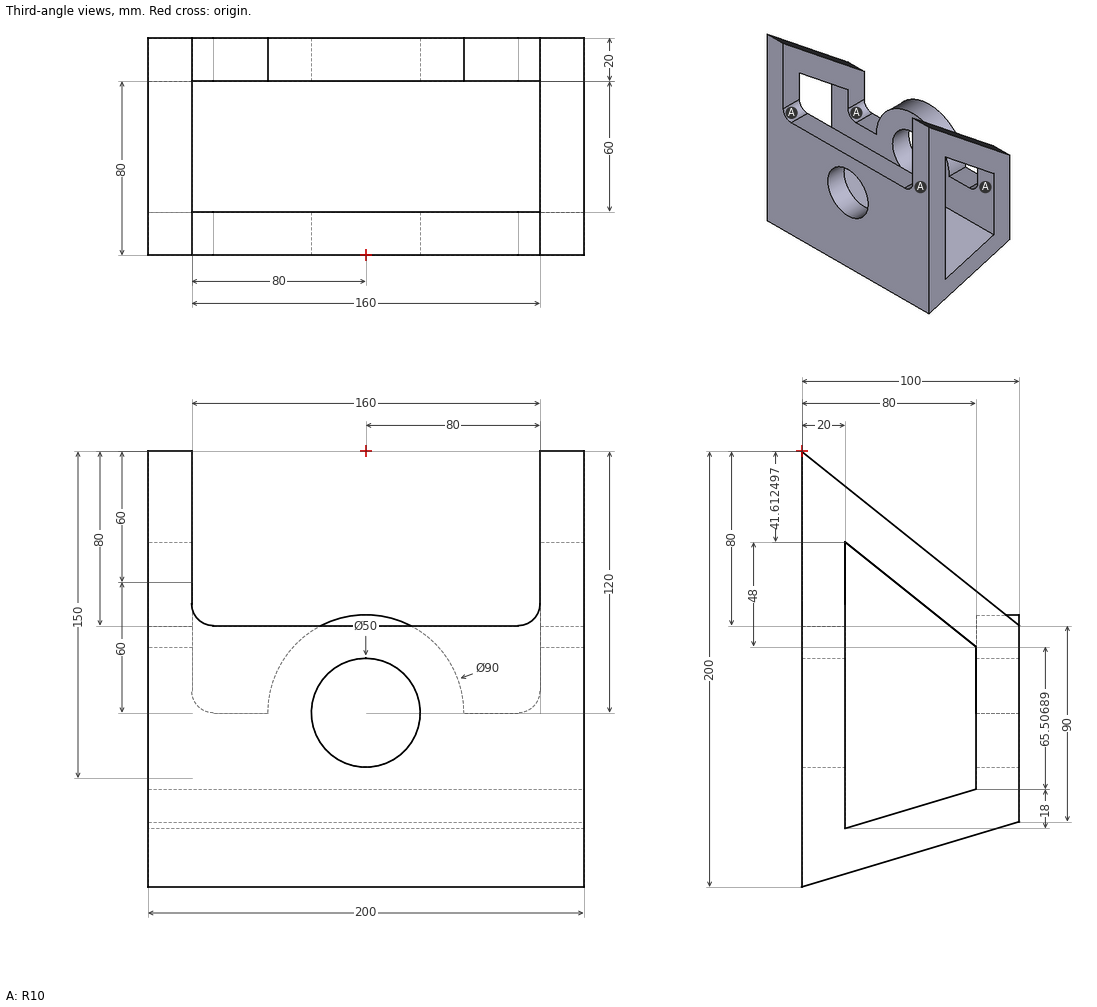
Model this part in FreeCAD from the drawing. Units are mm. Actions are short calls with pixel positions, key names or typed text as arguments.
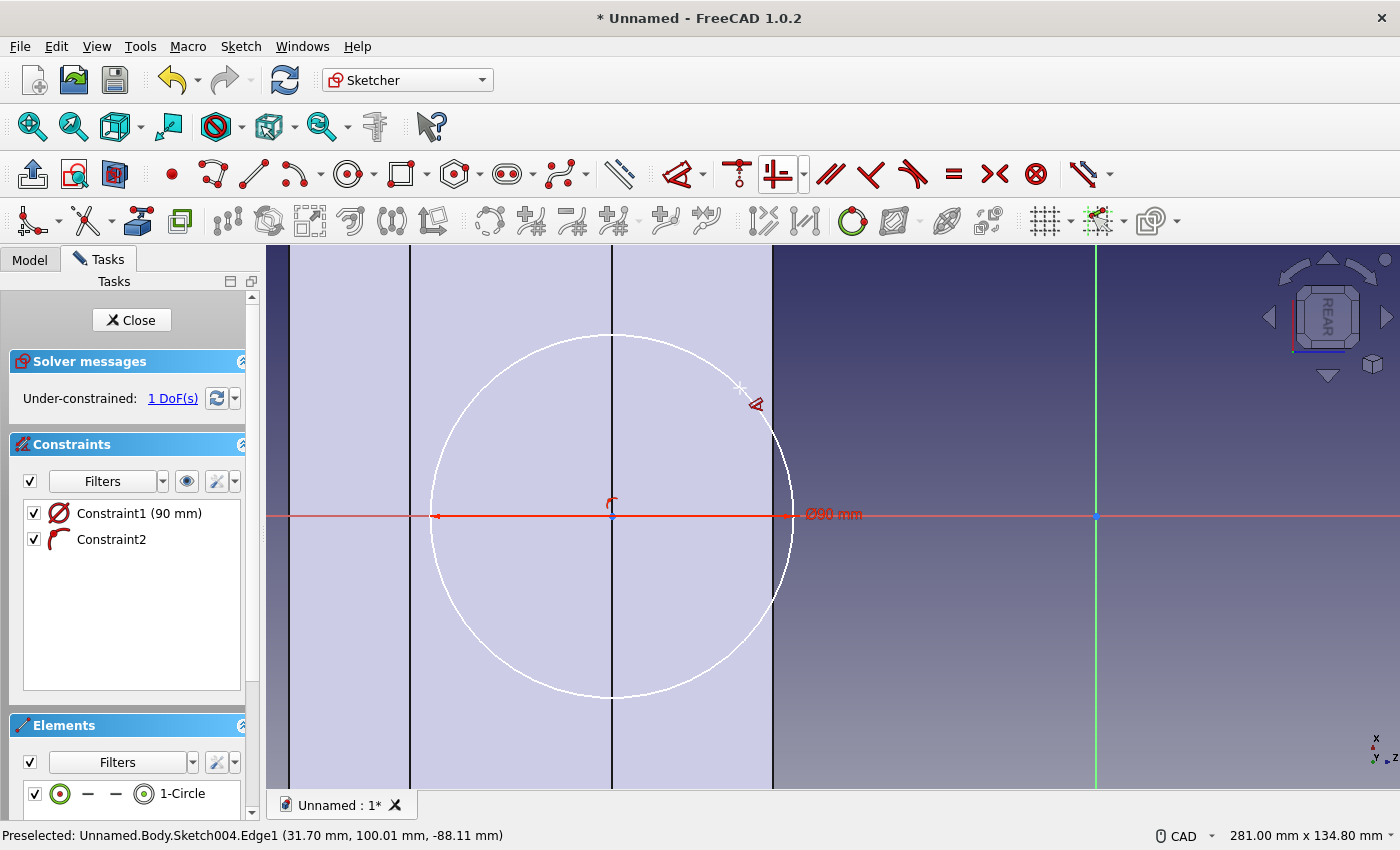
click(612, 516)
click(854, 550)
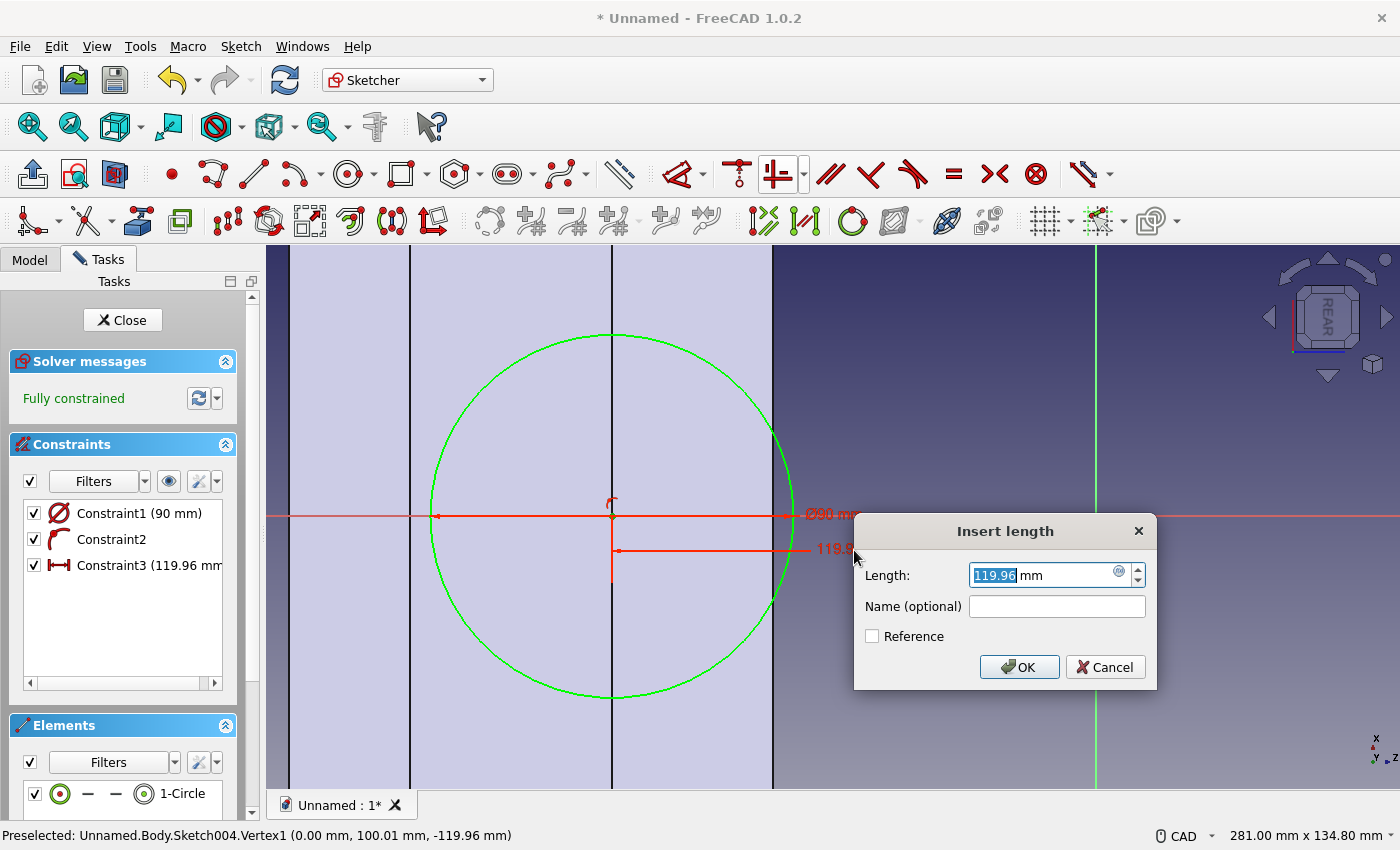
text(120)
key(Return)
key(Escape)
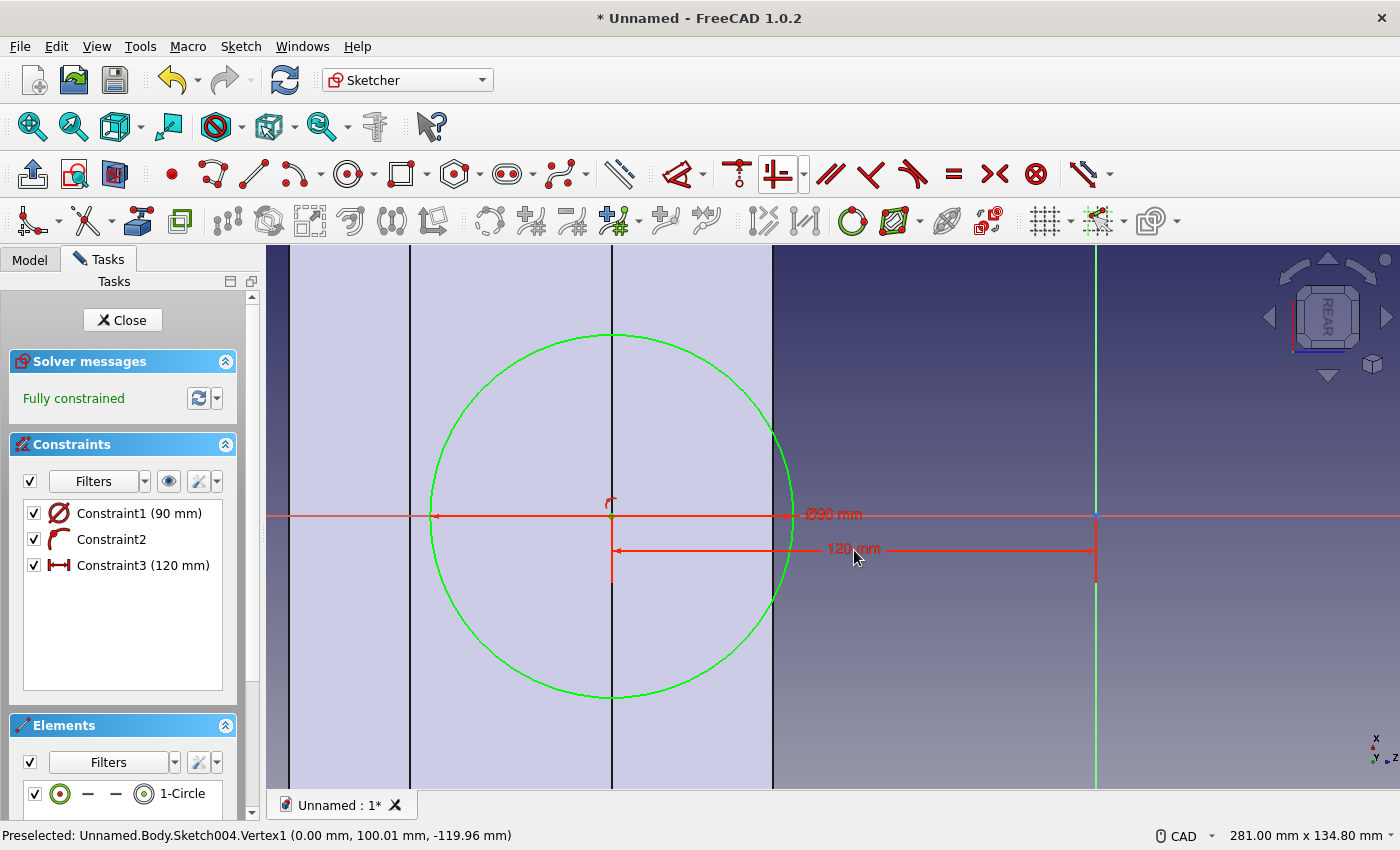
click(123, 320)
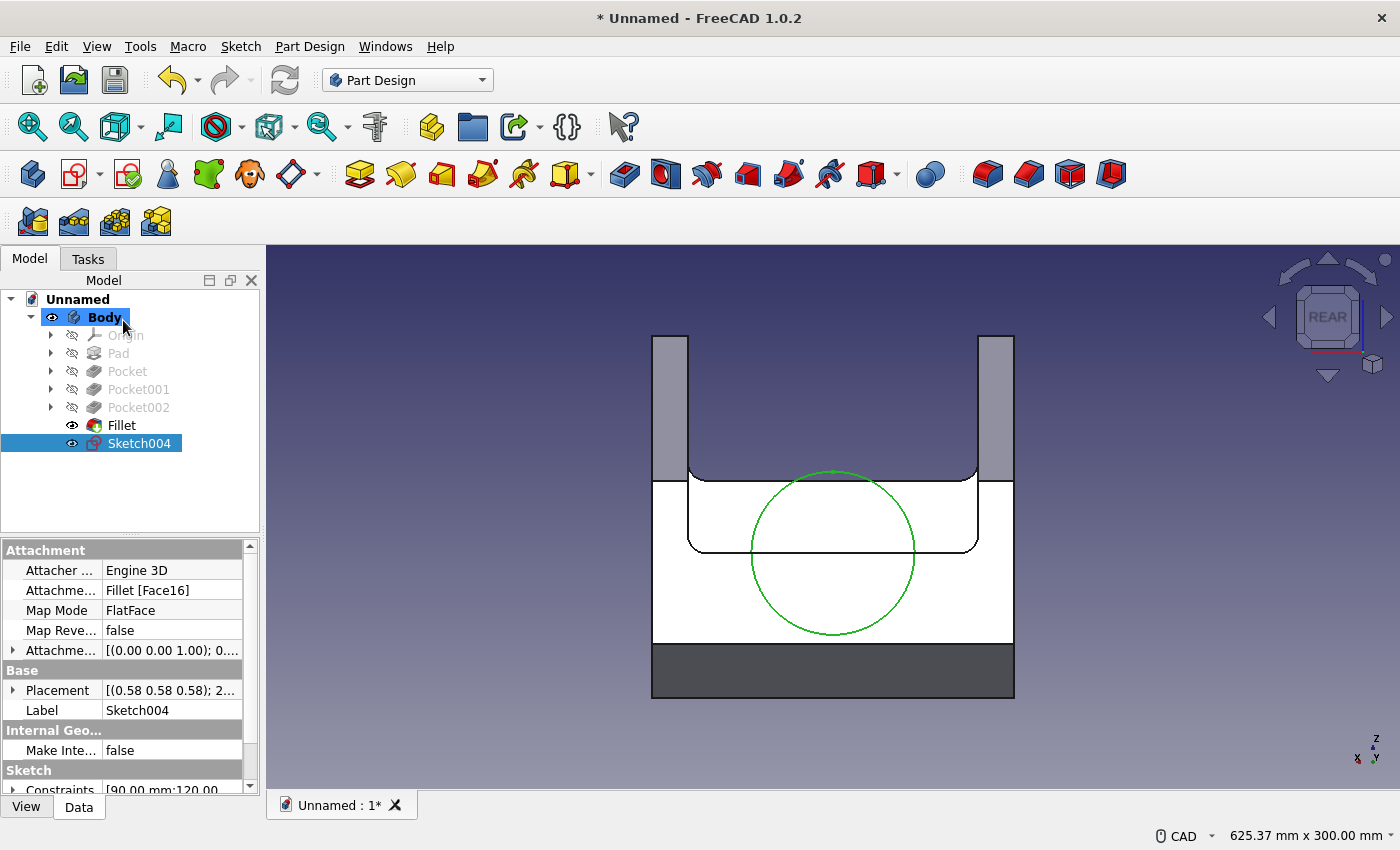
click(360, 174)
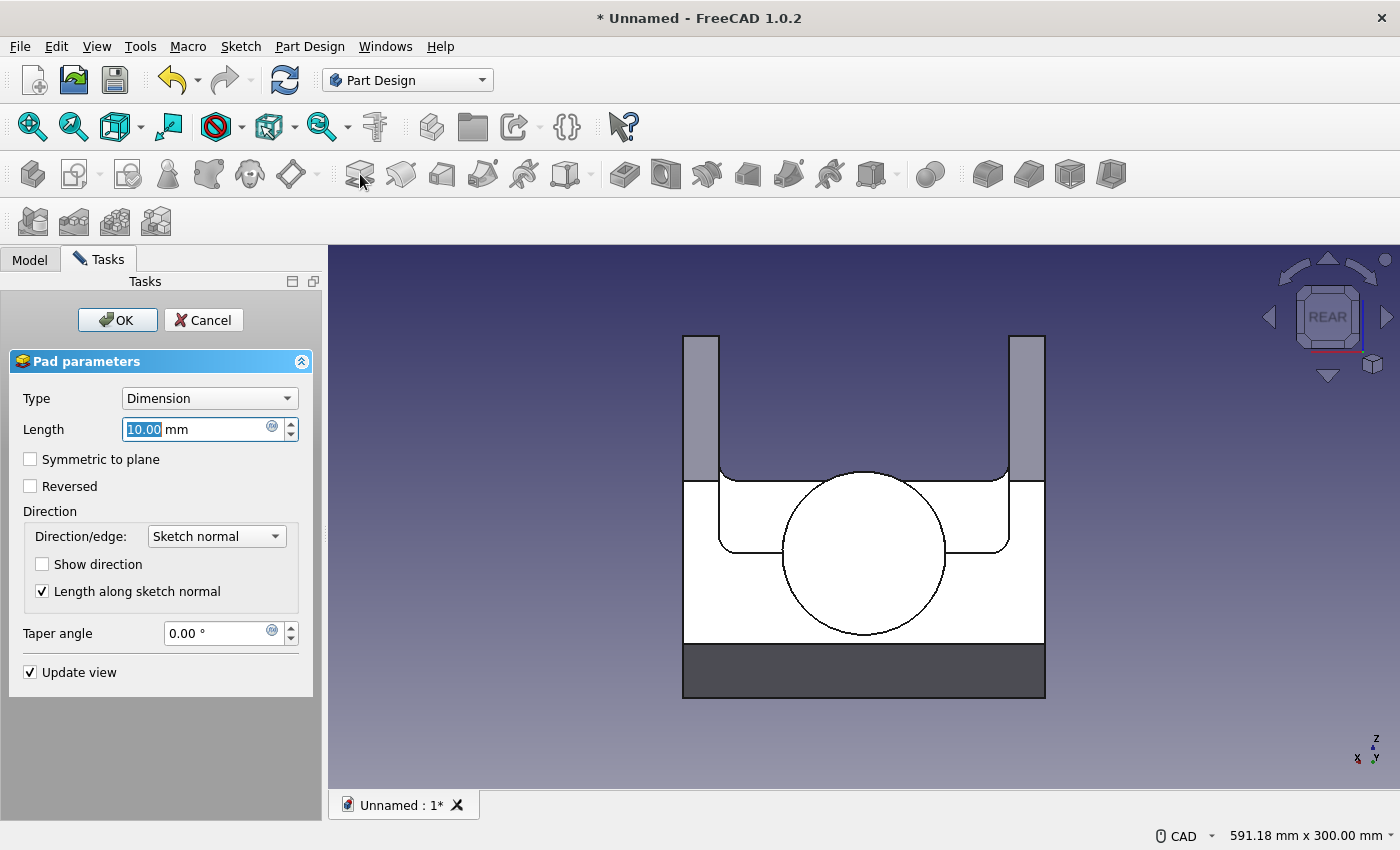
text(20)
key(Tab)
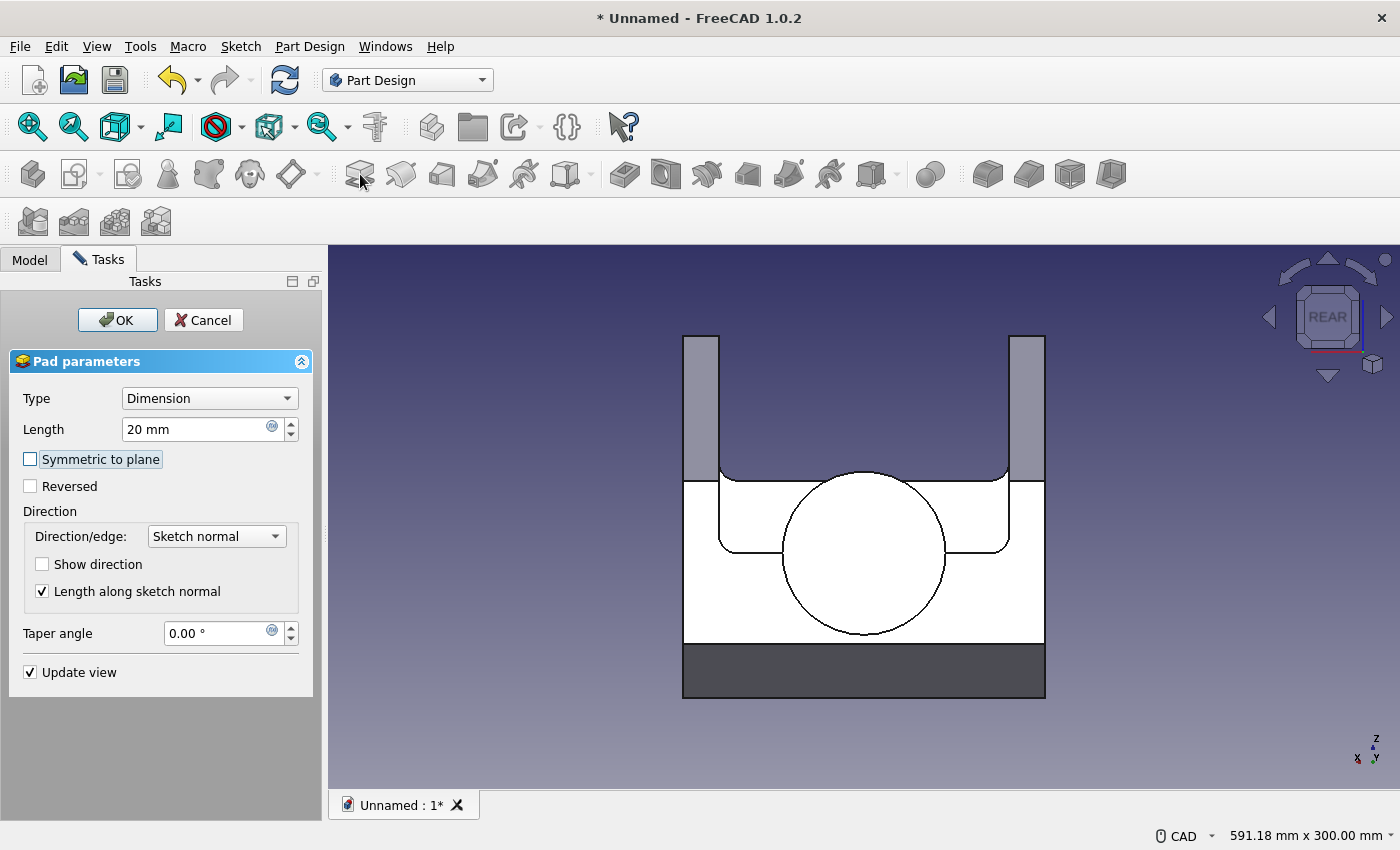
click(31, 486)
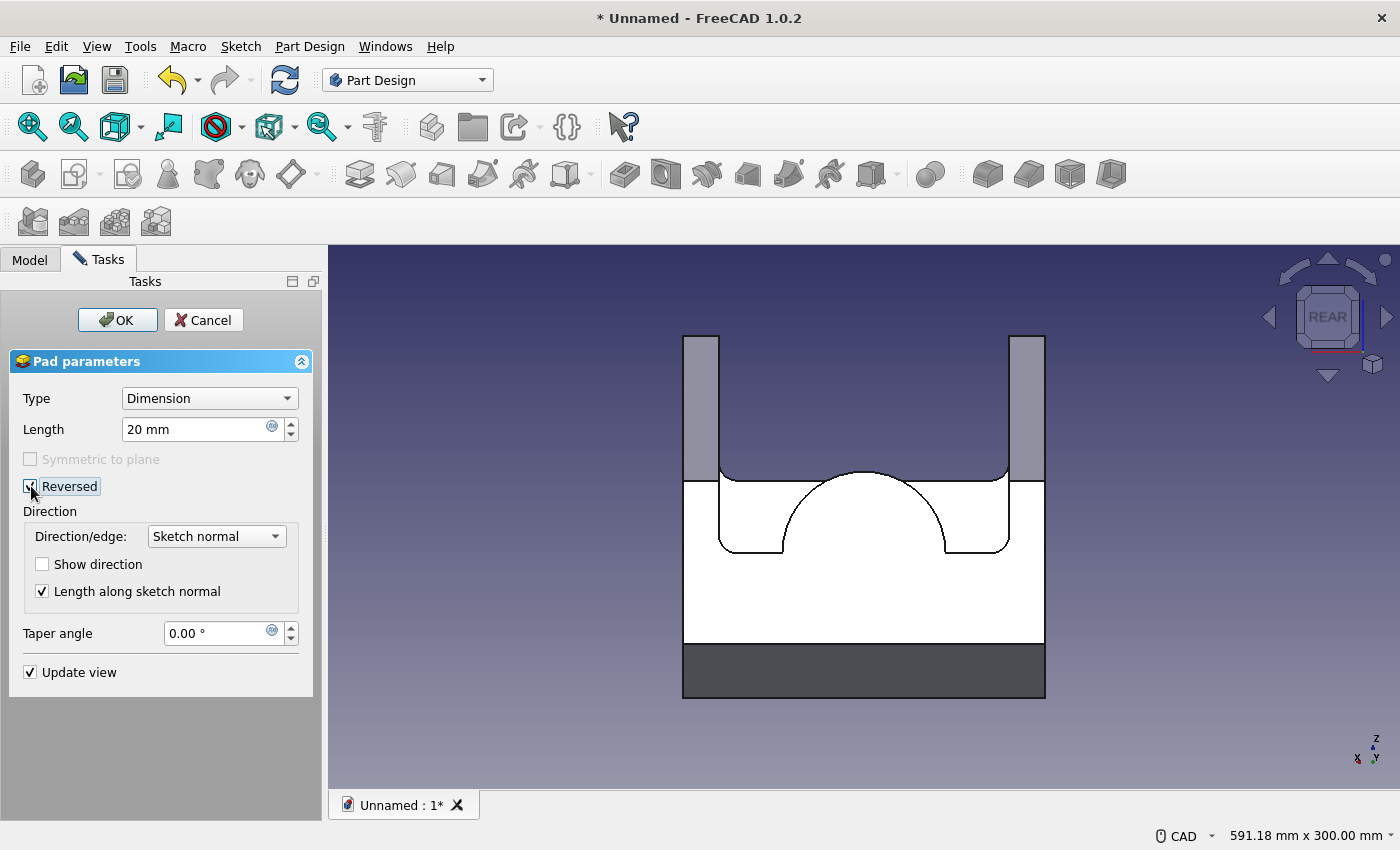
click(118, 320)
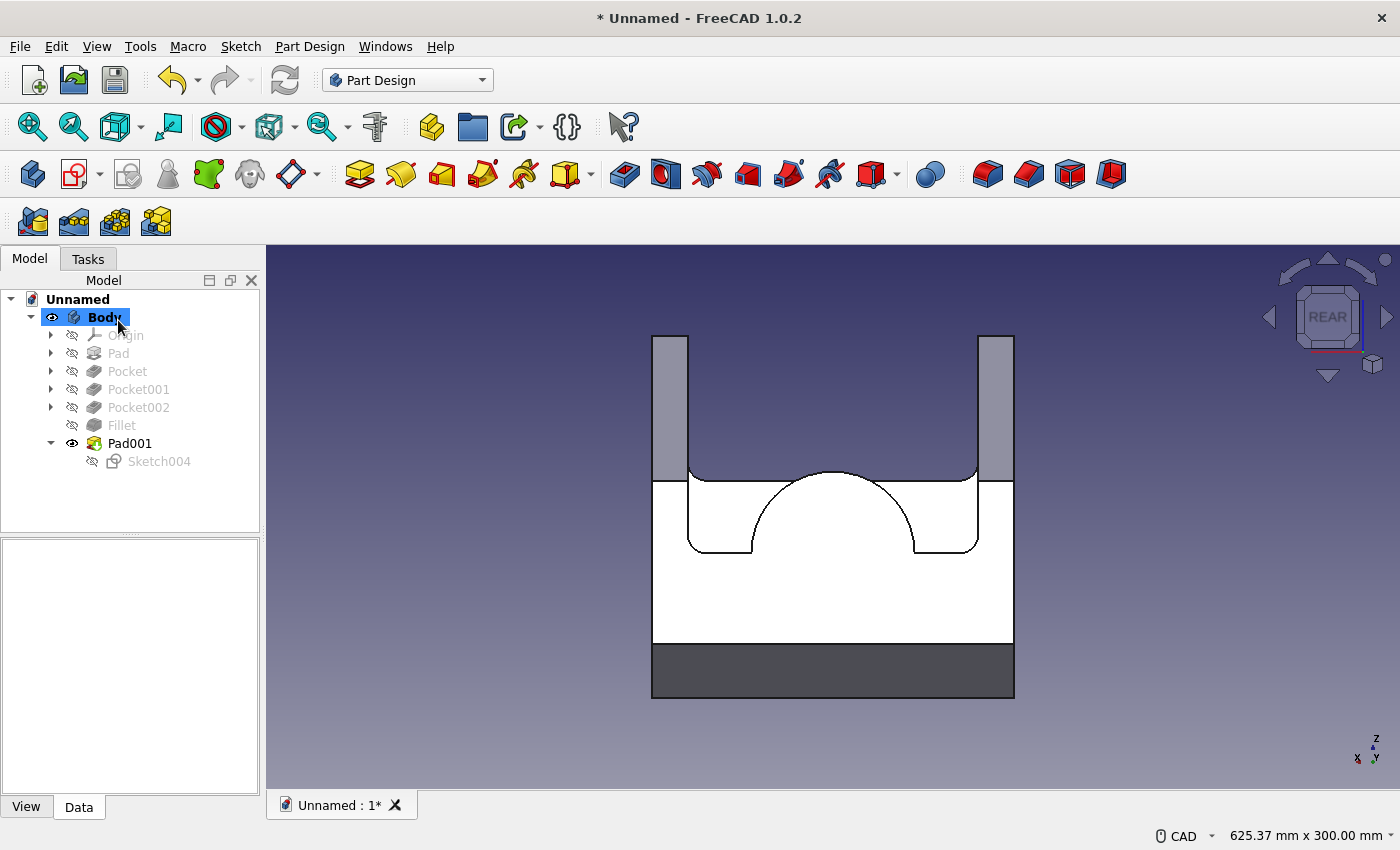
click(833, 557)